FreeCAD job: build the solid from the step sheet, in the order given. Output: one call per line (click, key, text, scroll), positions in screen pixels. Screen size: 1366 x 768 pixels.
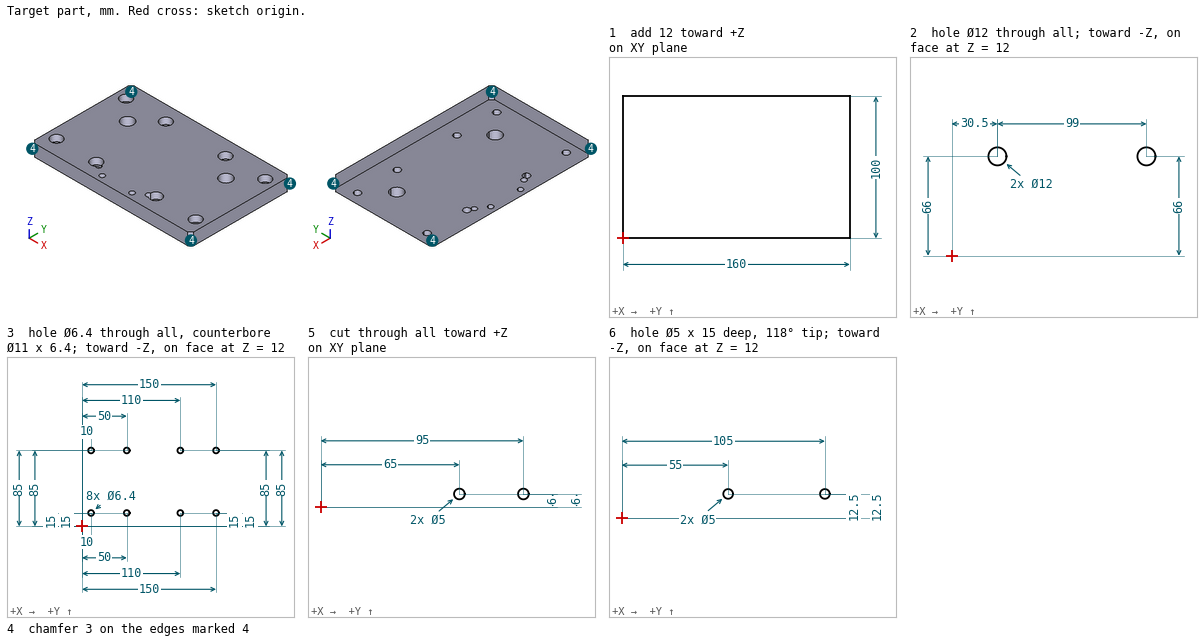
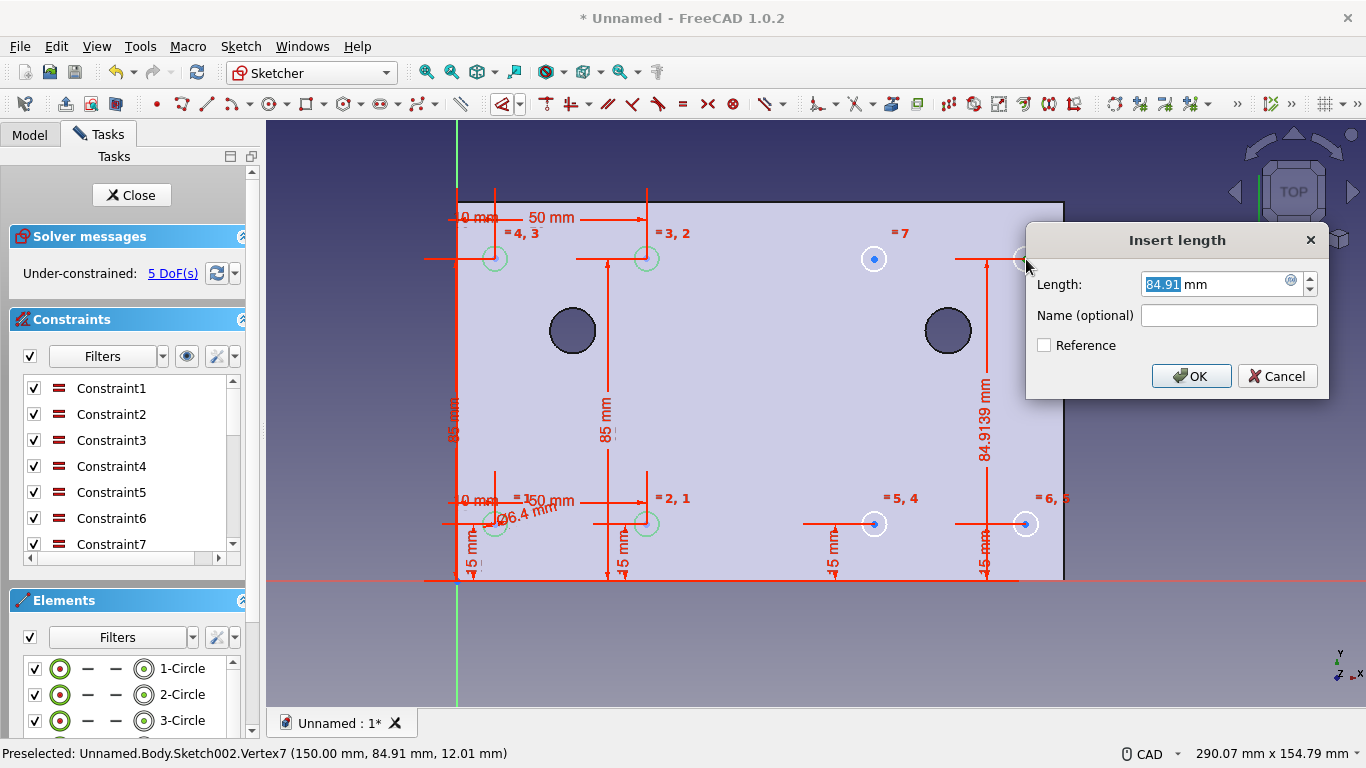
text(85)
key(Return)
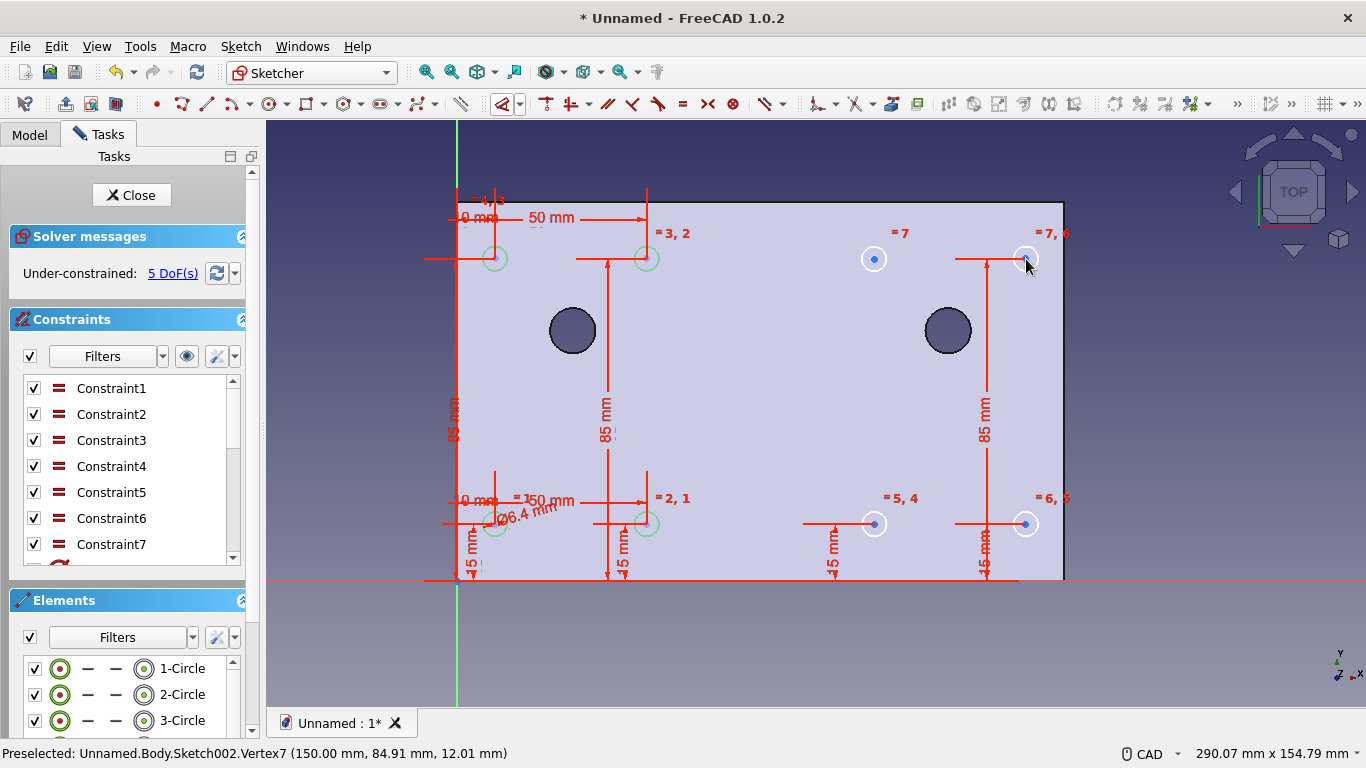
click(874, 259)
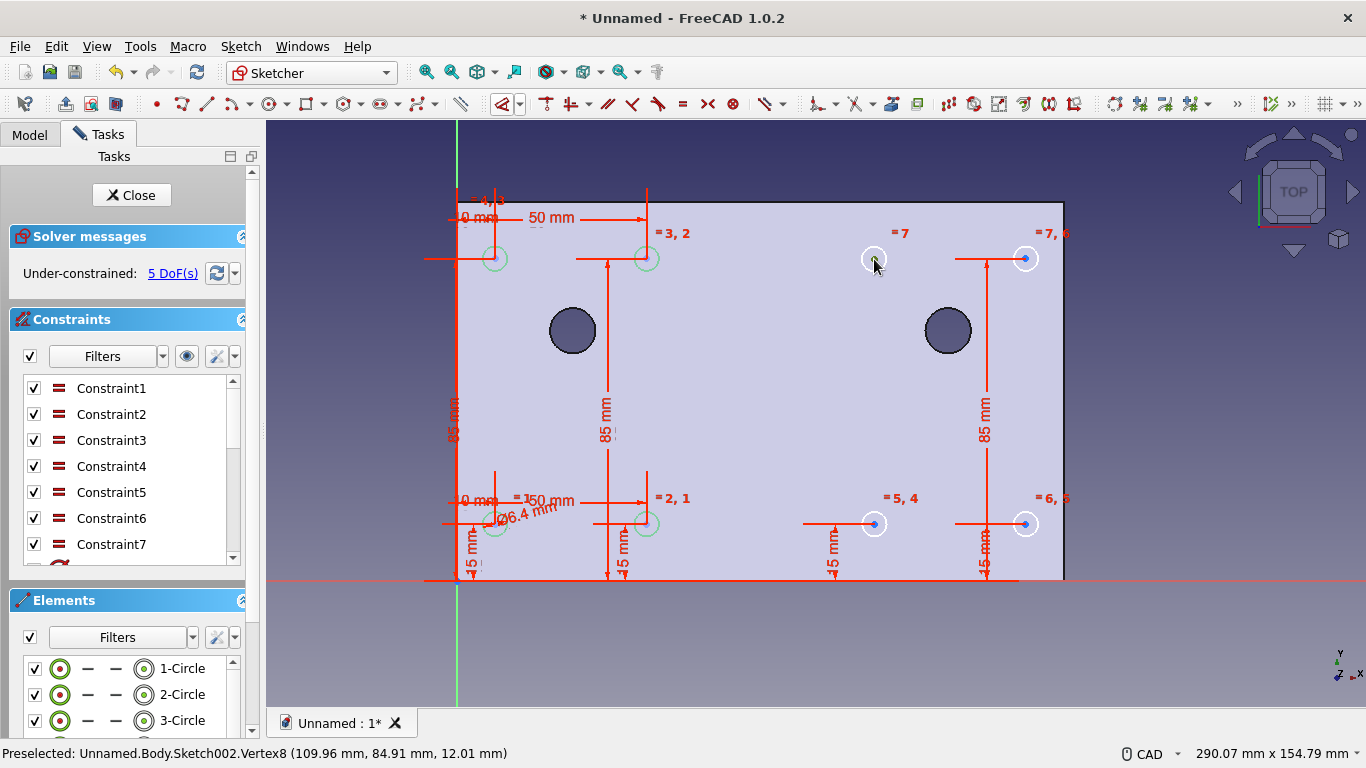
key(i)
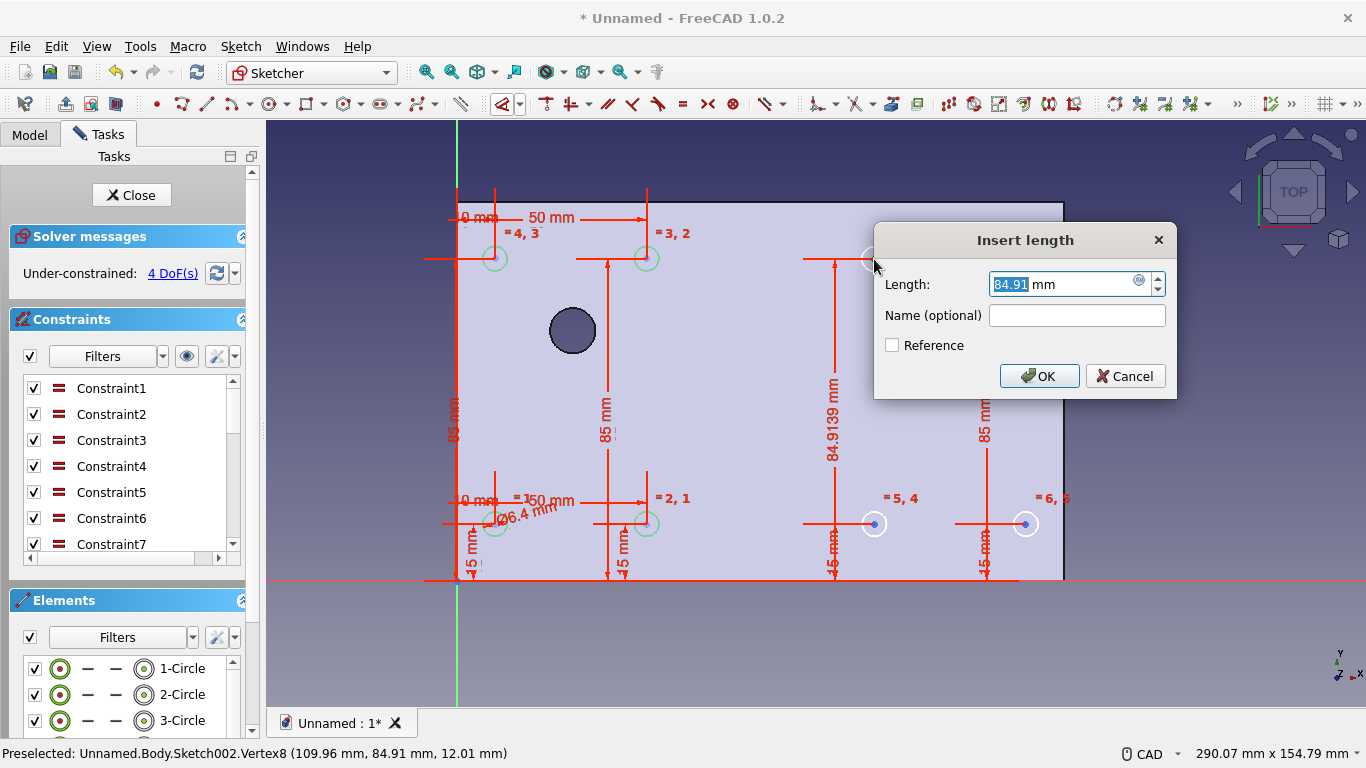
text(85)
key(Return)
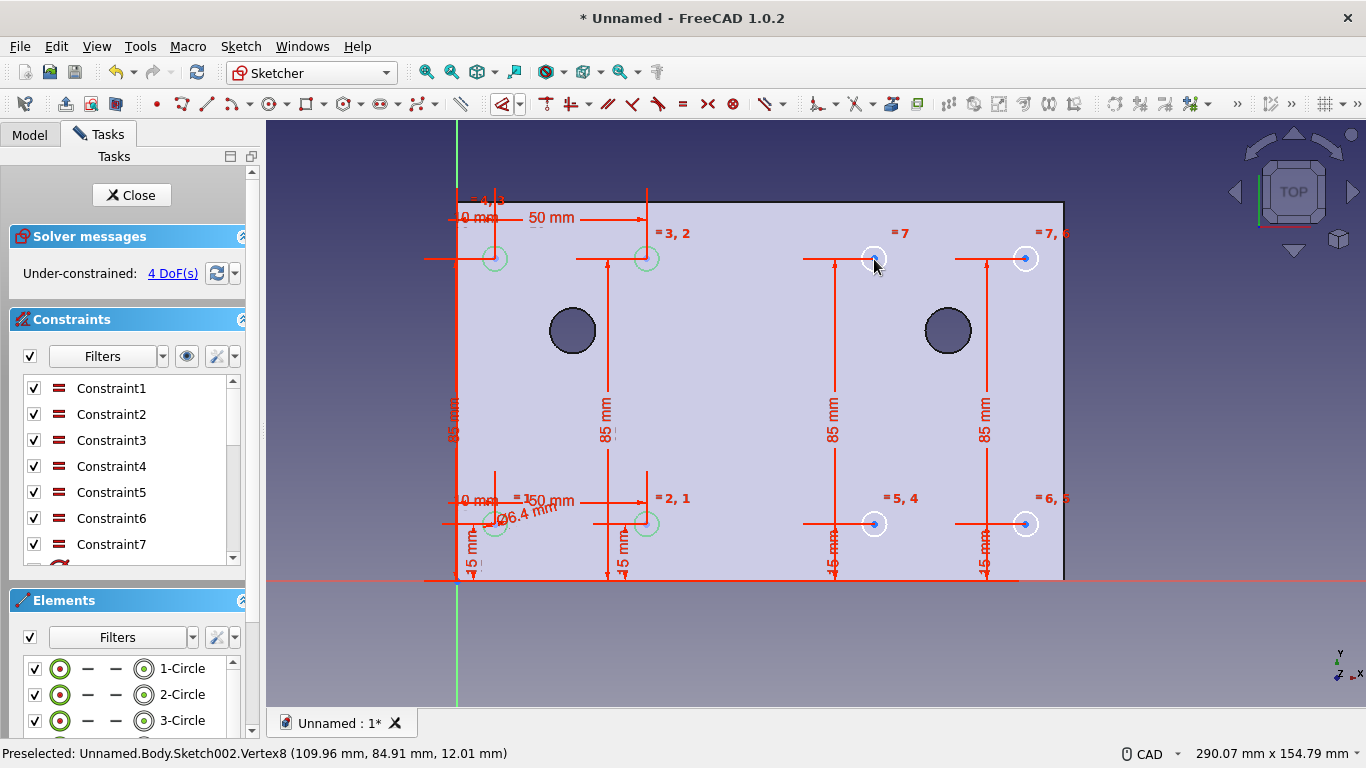
click(874, 524)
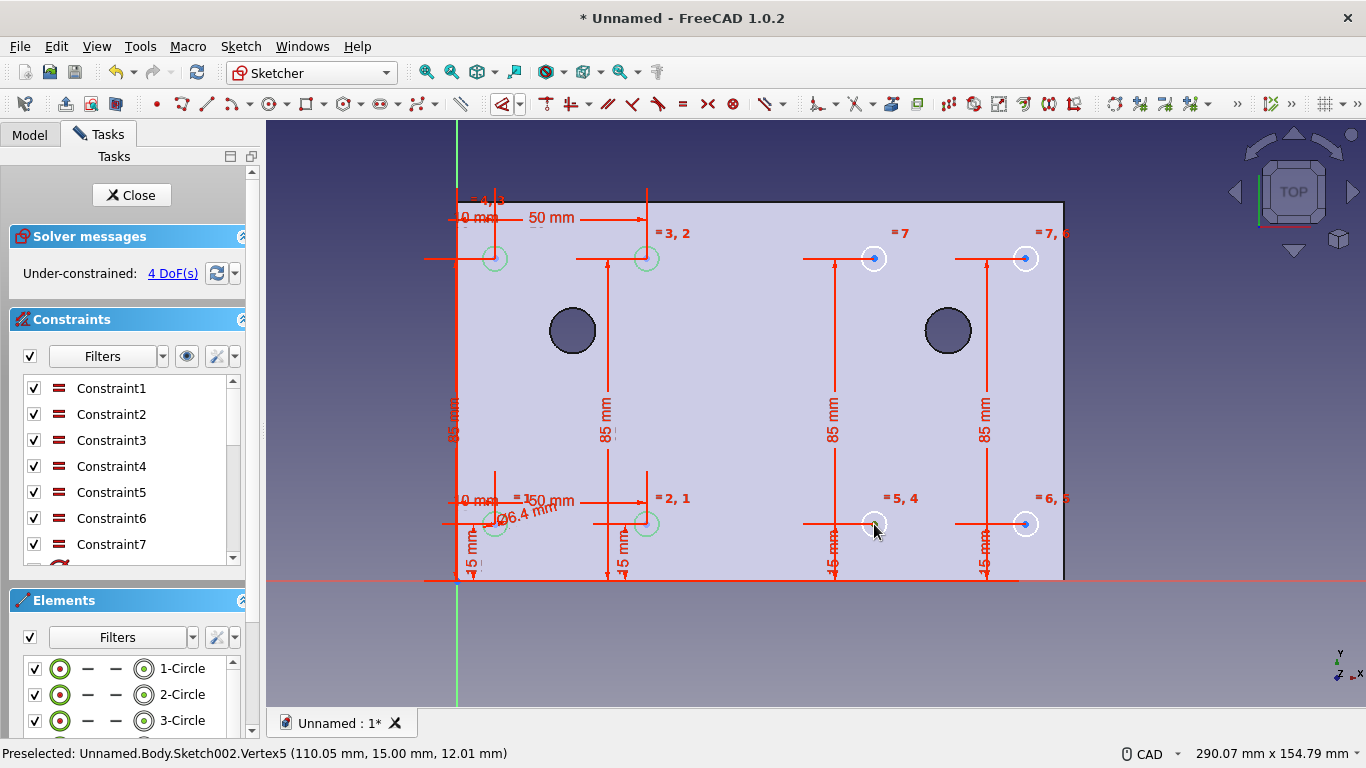
key(l)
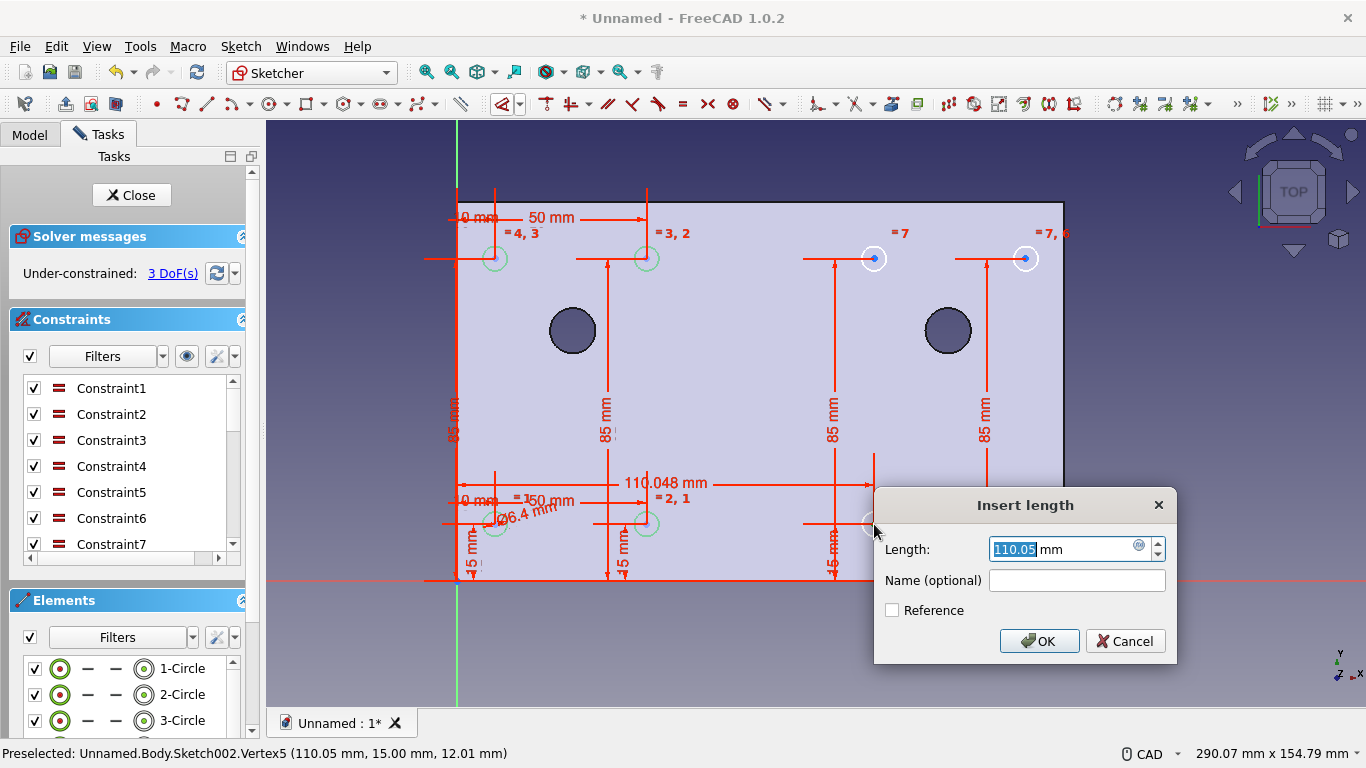
text(110)
key(Return)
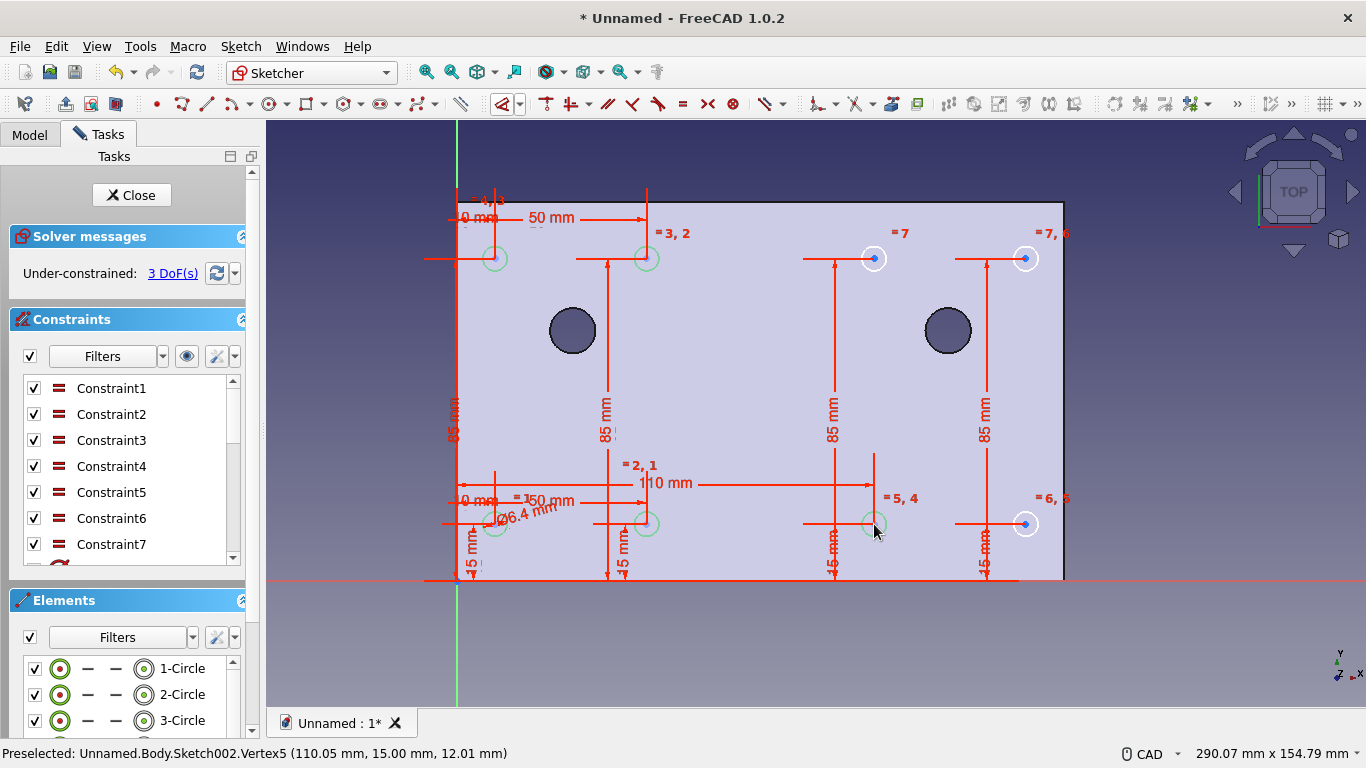
click(1026, 524)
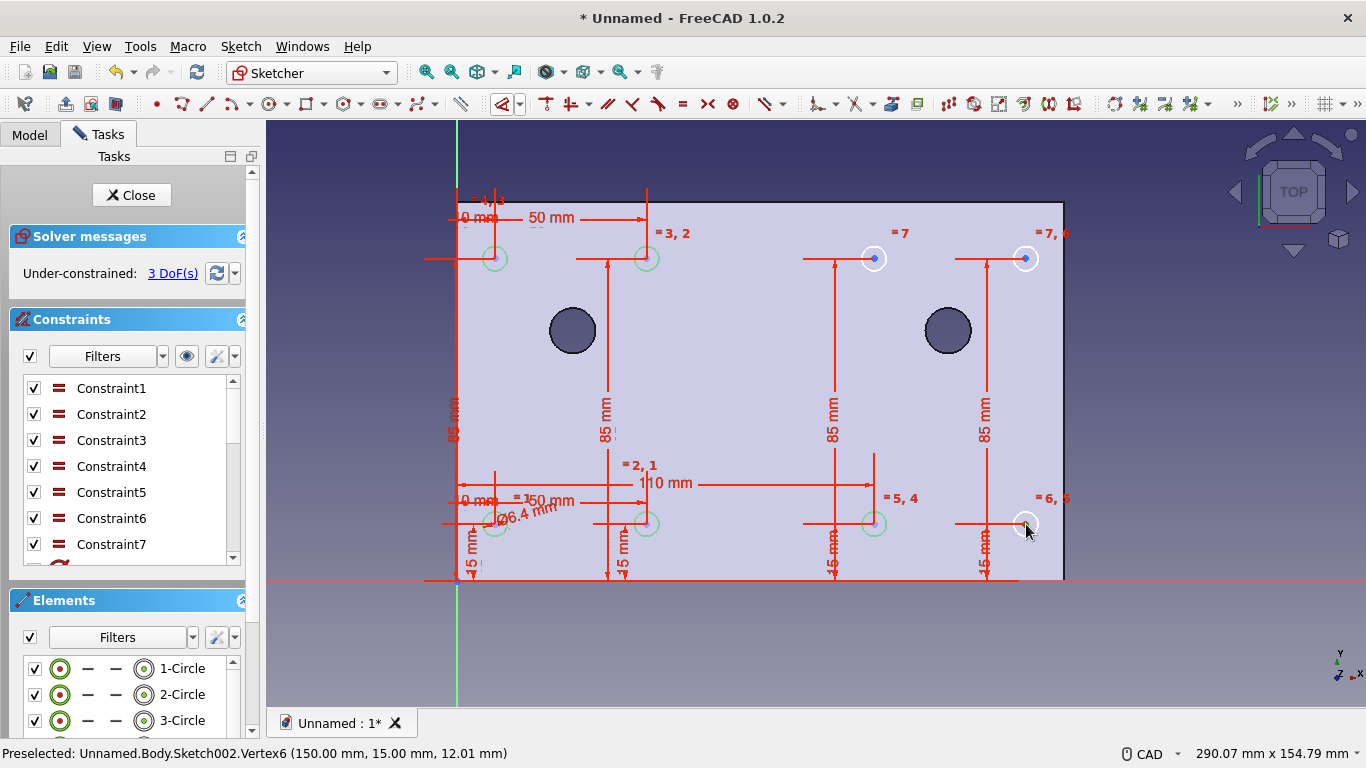
click(520, 104)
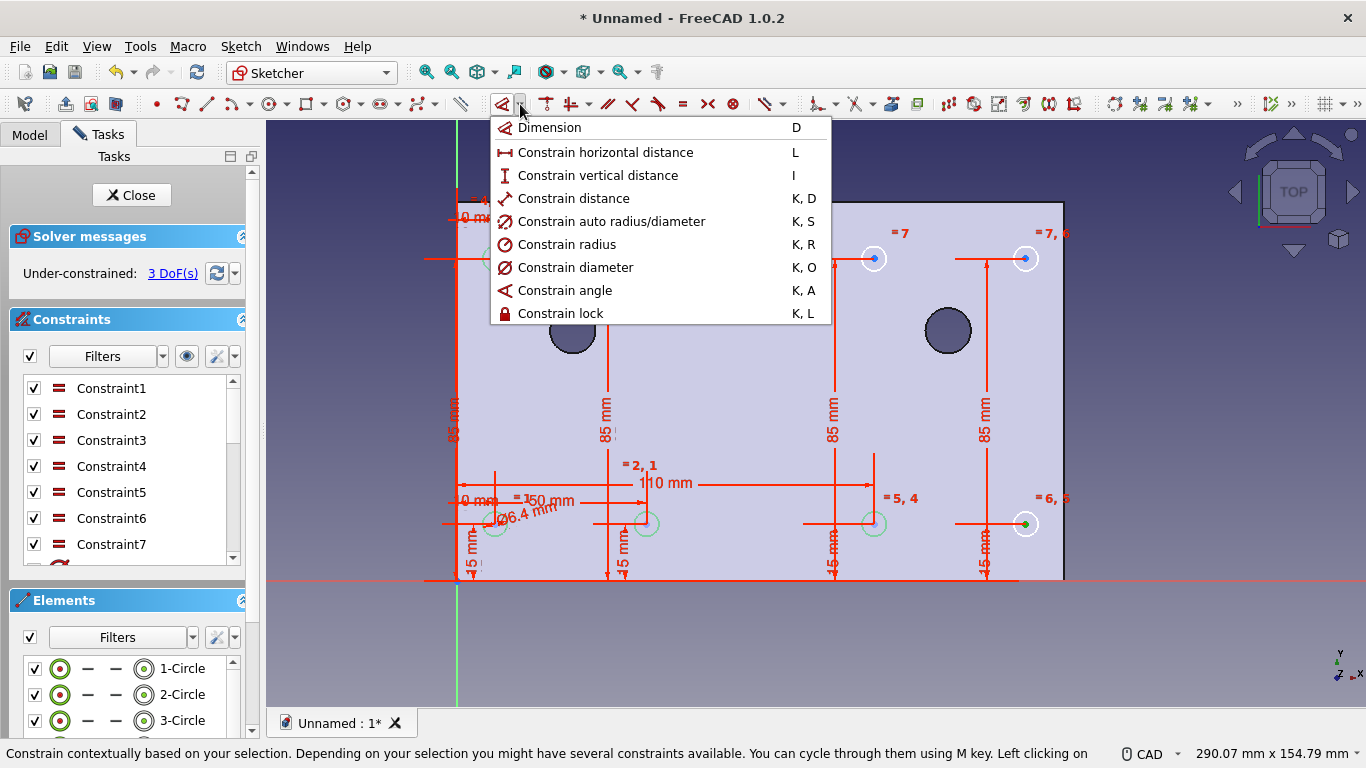
click(661, 152)